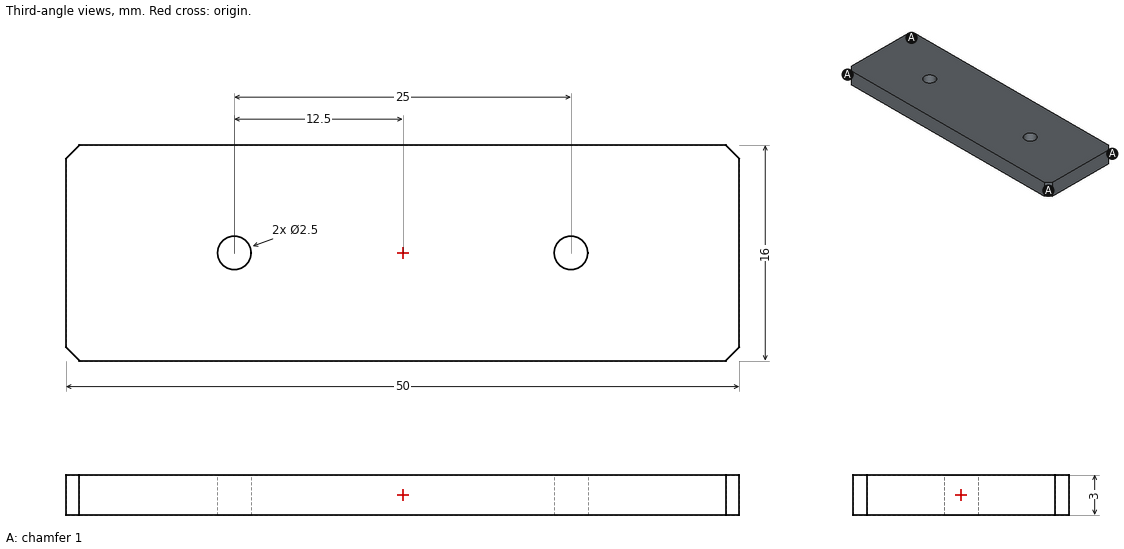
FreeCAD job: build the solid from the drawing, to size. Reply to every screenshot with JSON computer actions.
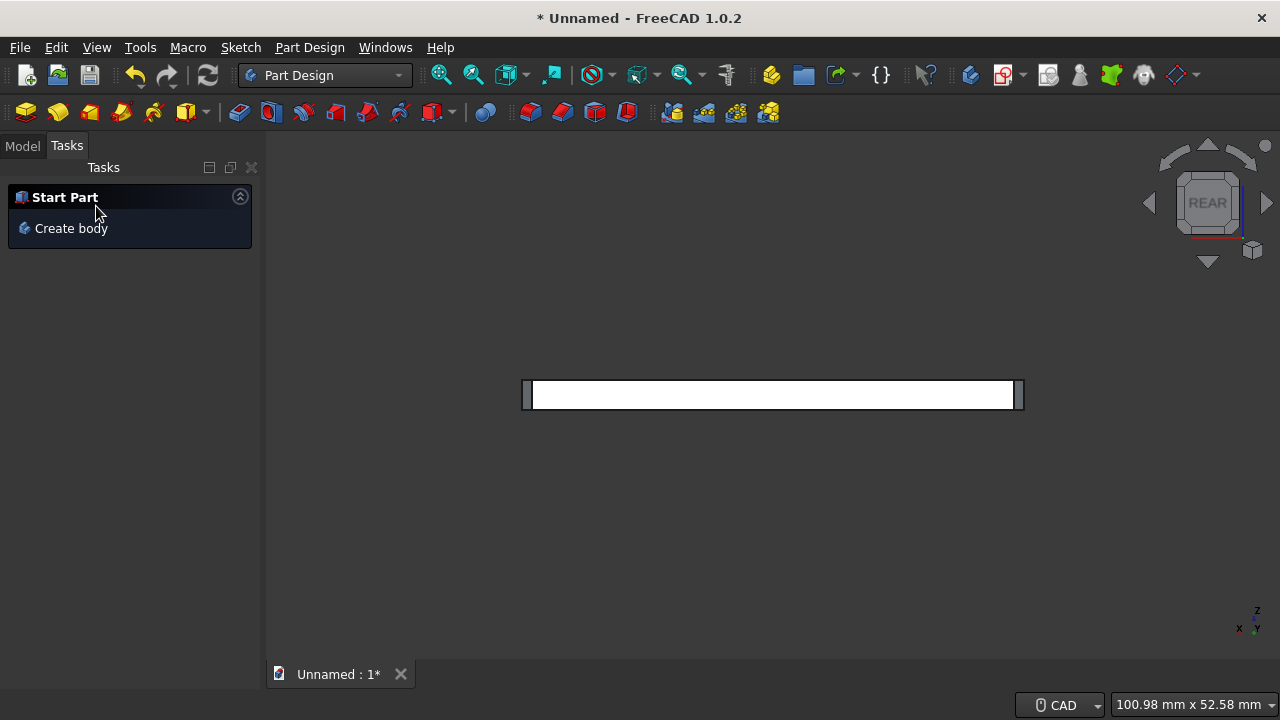
{"action": "key", "text": "0"}